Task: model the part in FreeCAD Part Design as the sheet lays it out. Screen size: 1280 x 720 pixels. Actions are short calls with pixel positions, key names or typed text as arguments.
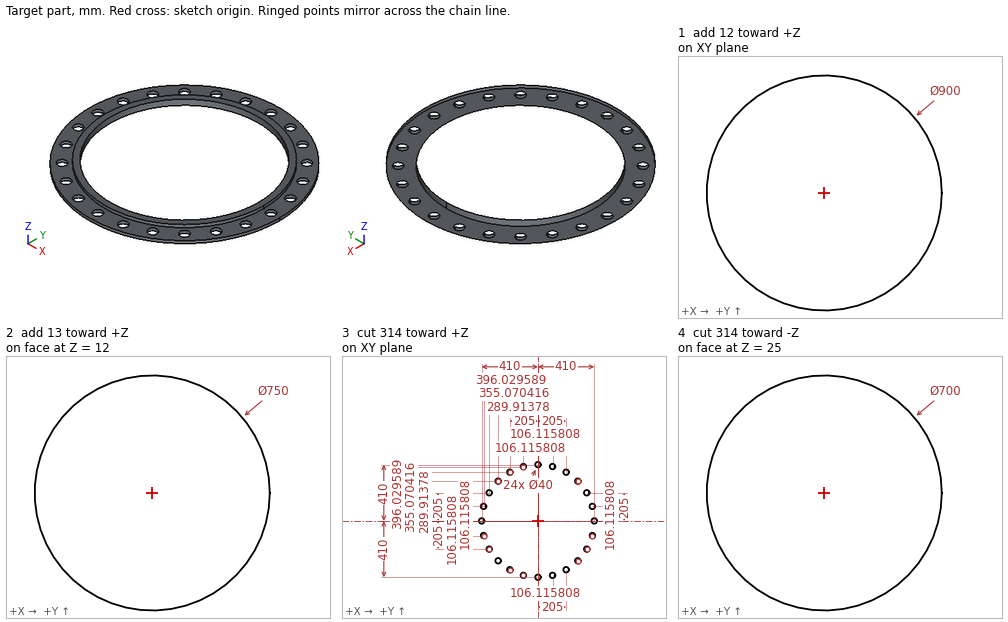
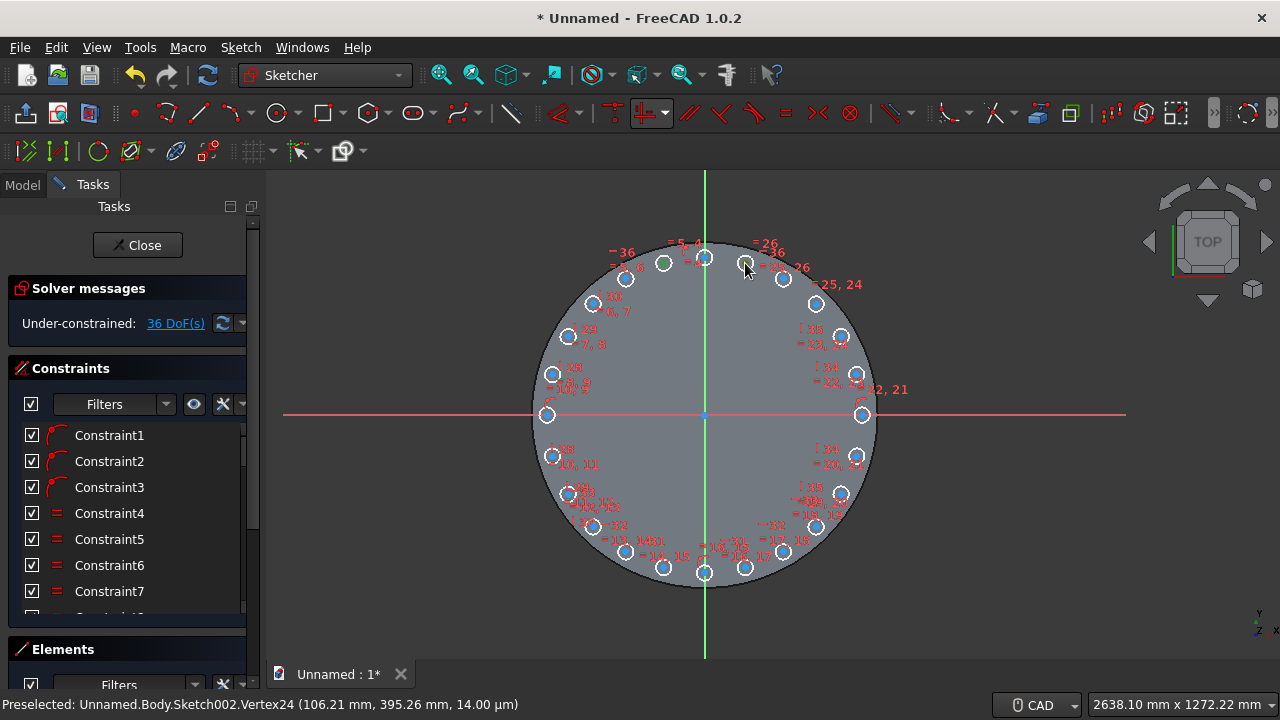
click(668, 114)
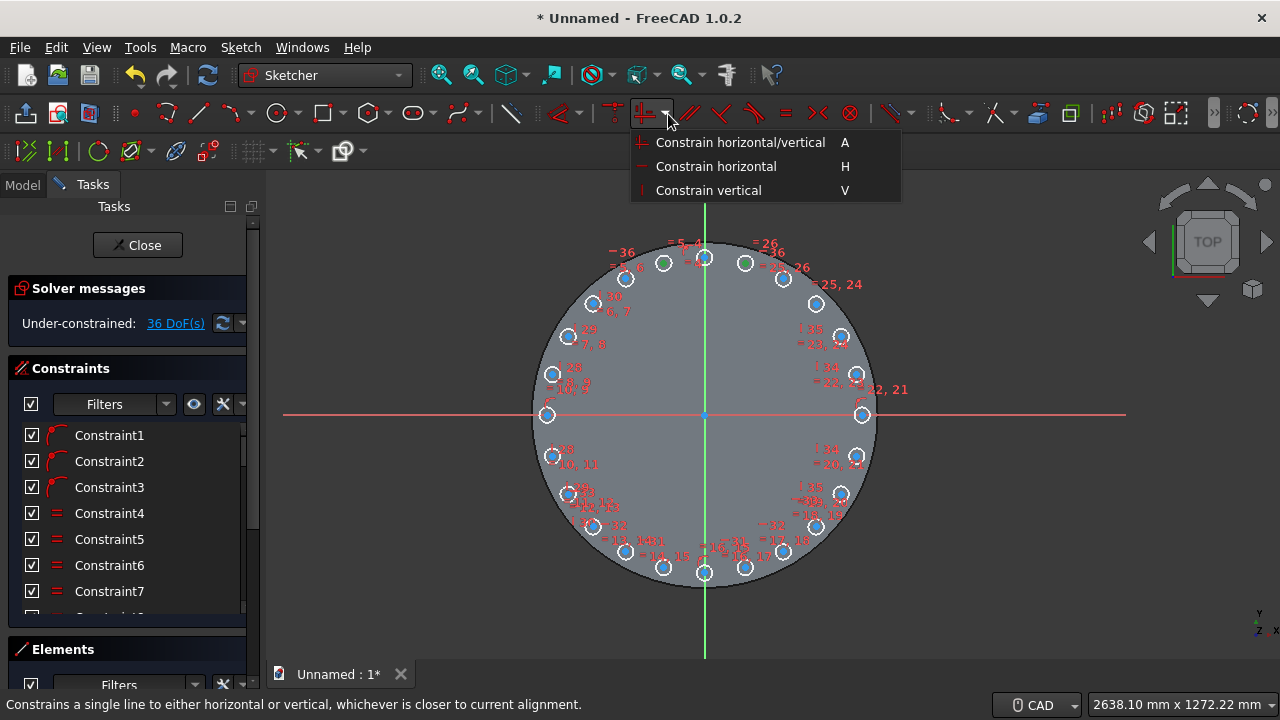
click(766, 166)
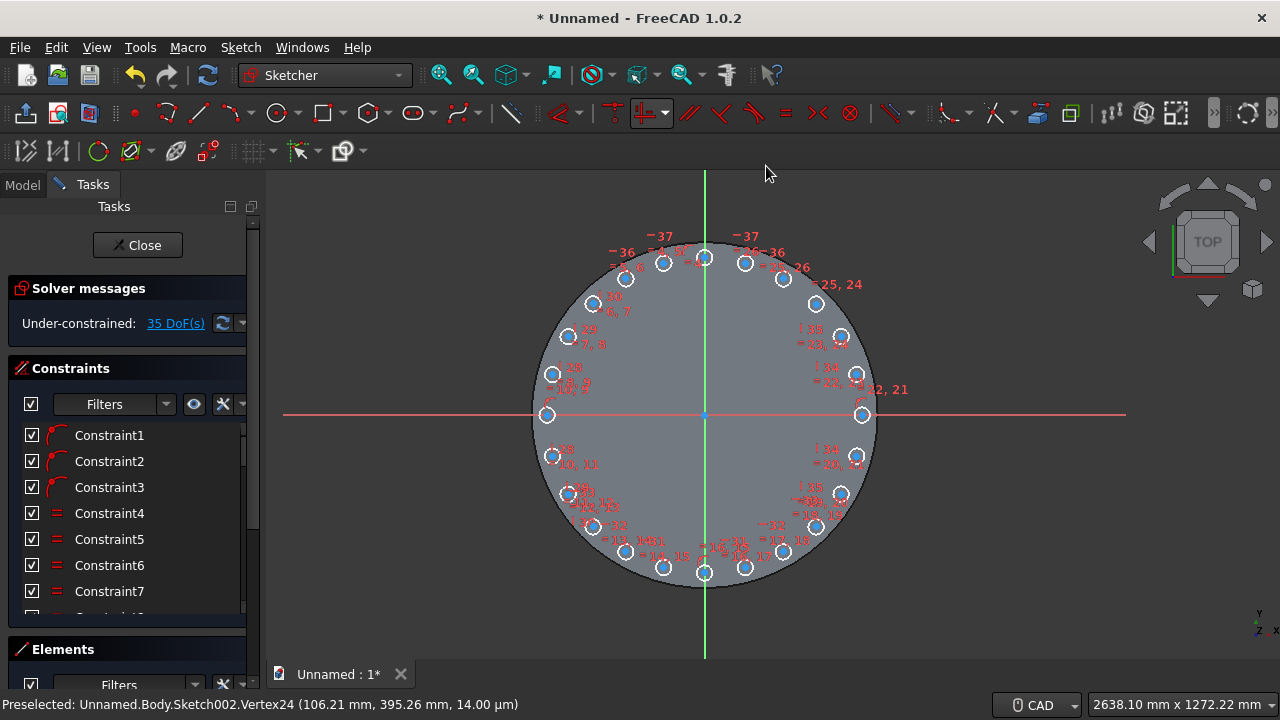
click(626, 279)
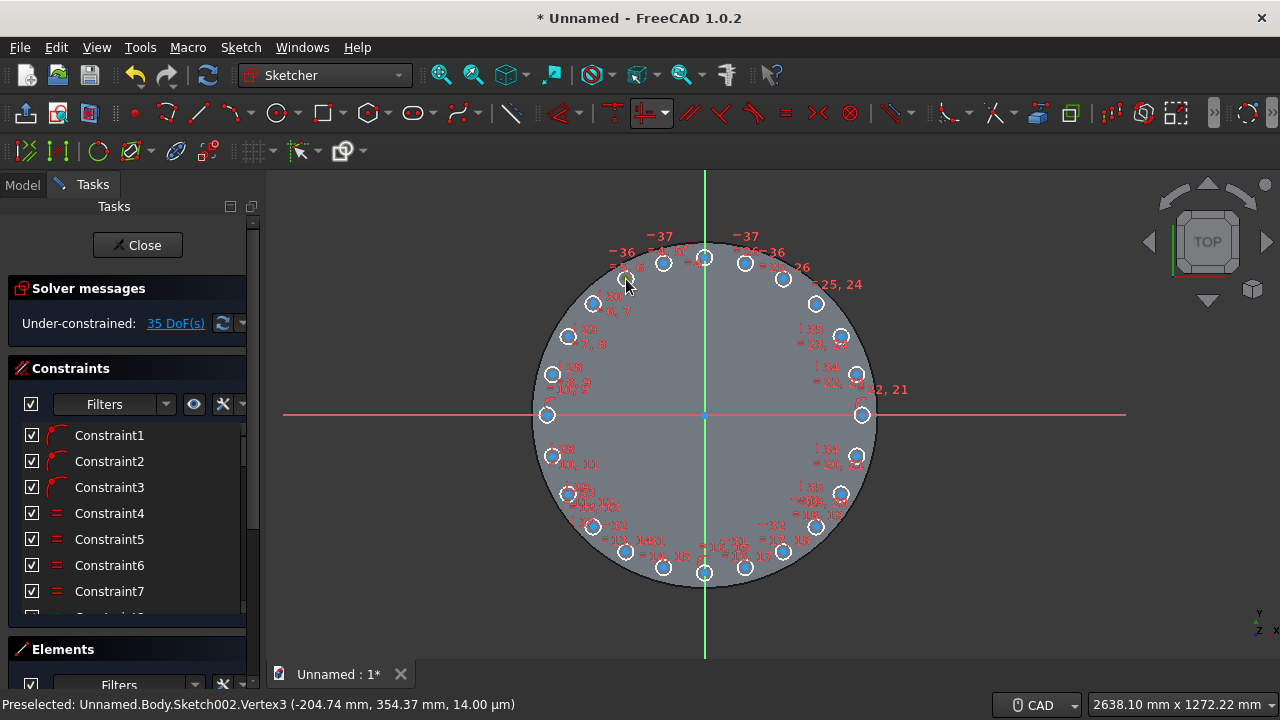
click(626, 552)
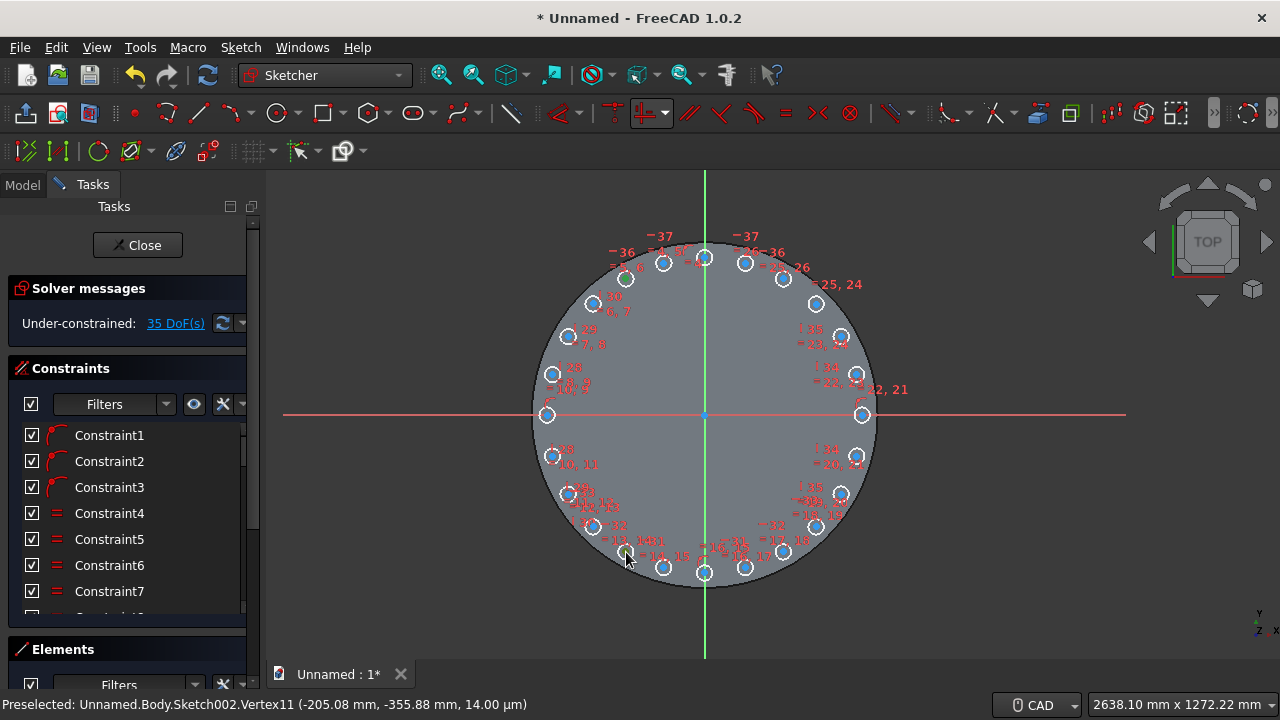
click(353, 415)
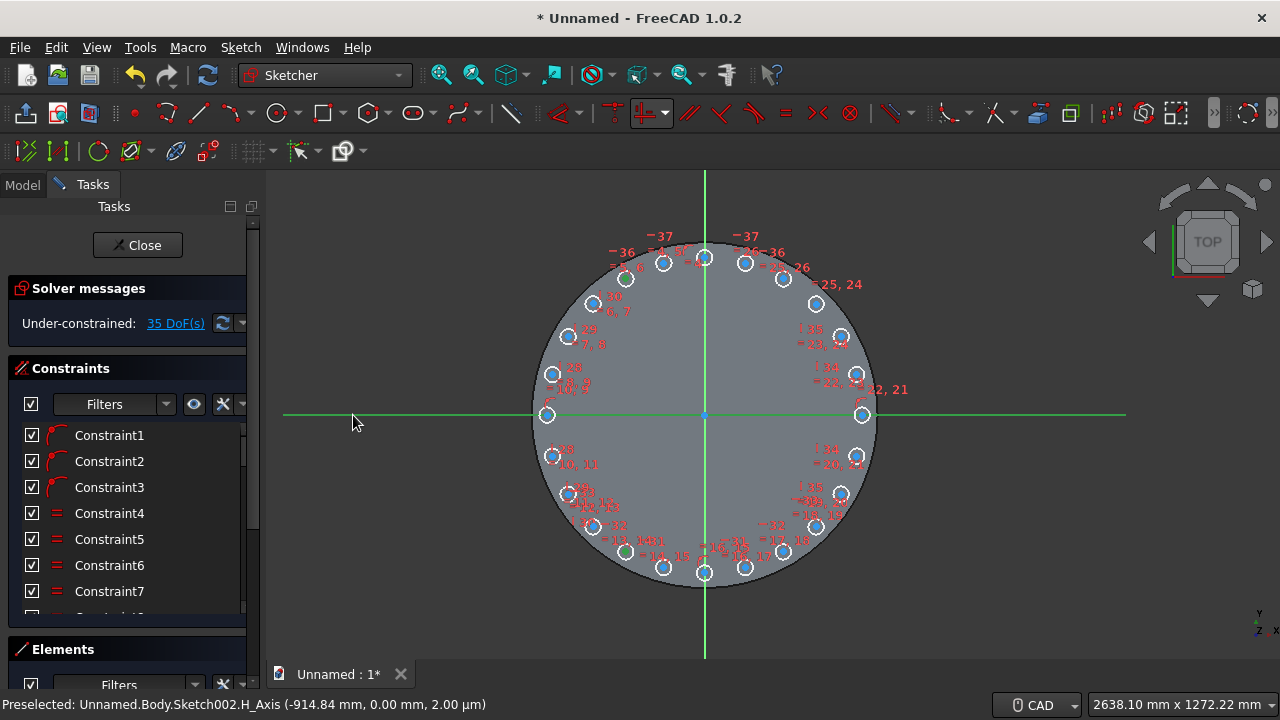
click(818, 114)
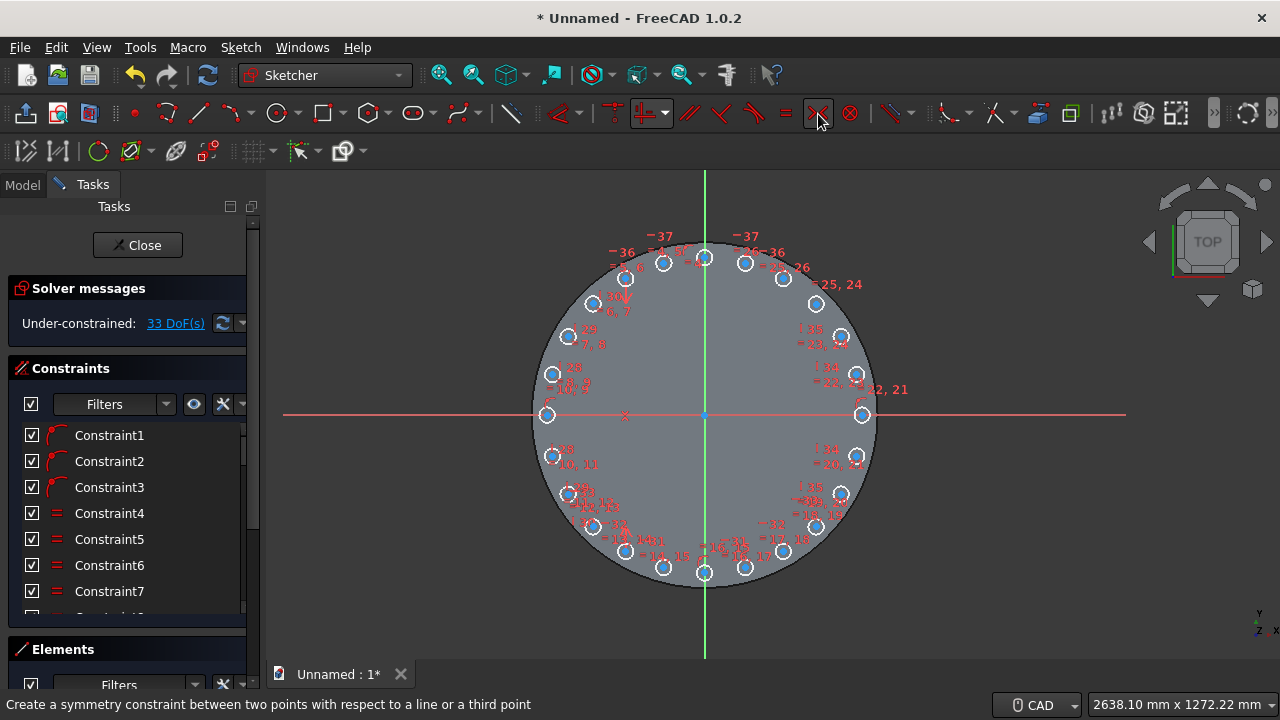
click(664, 263)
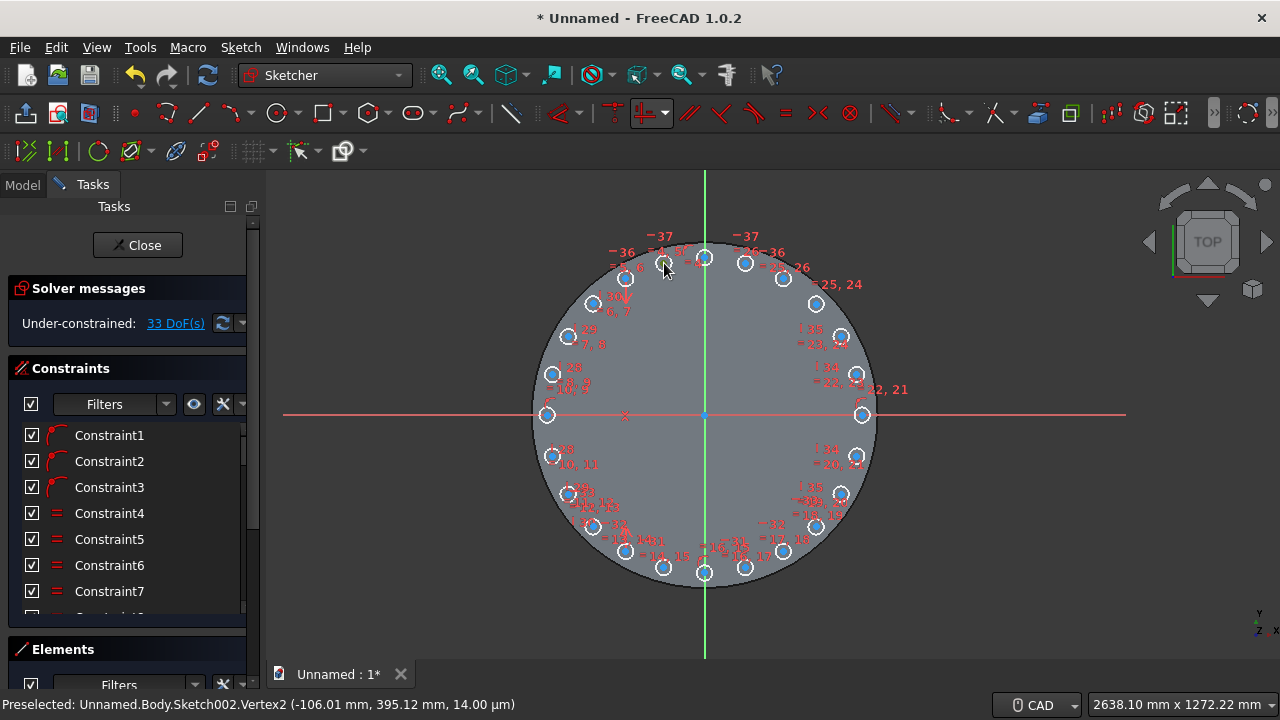
click(664, 568)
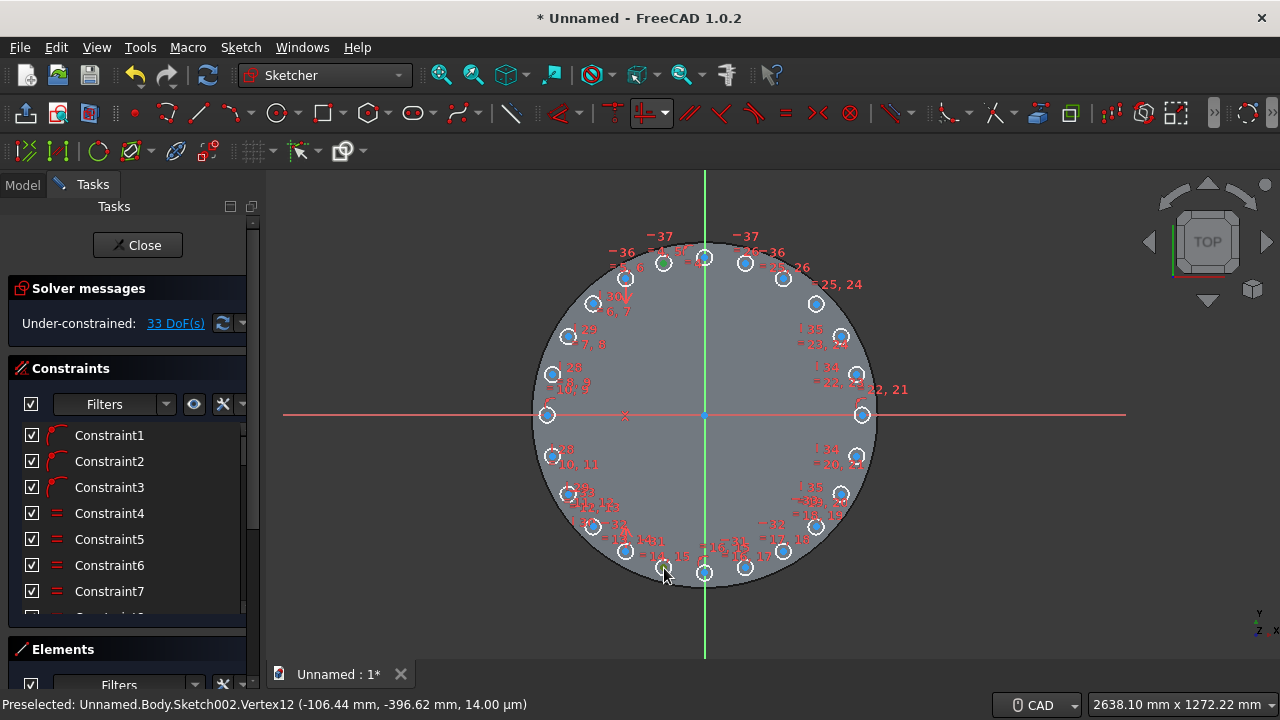
click(353, 415)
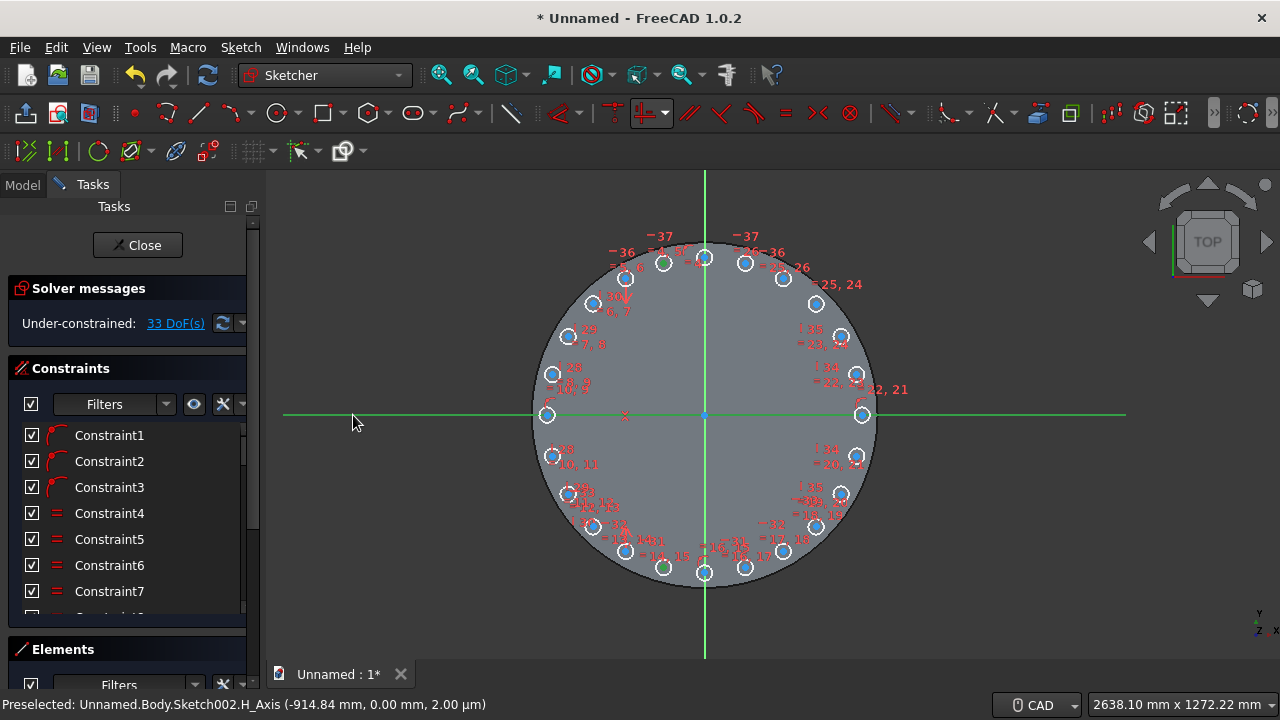
click(818, 114)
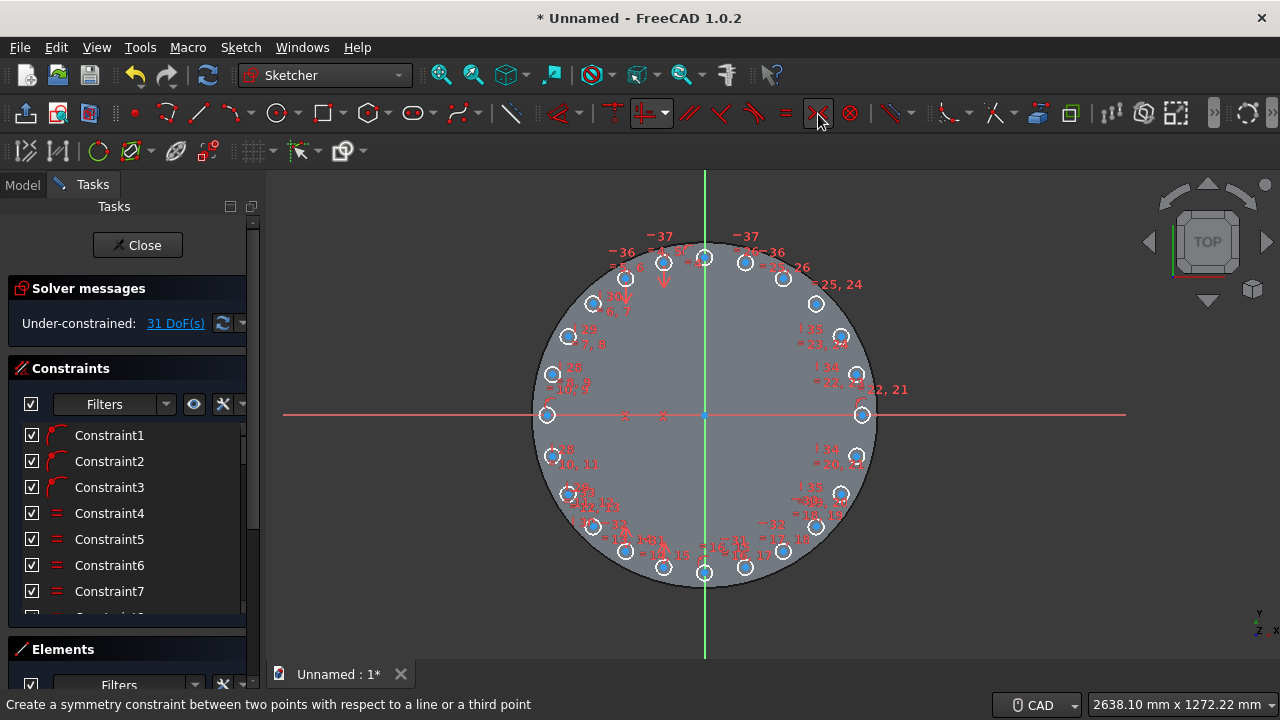
scroll(568, 494, up, 4)